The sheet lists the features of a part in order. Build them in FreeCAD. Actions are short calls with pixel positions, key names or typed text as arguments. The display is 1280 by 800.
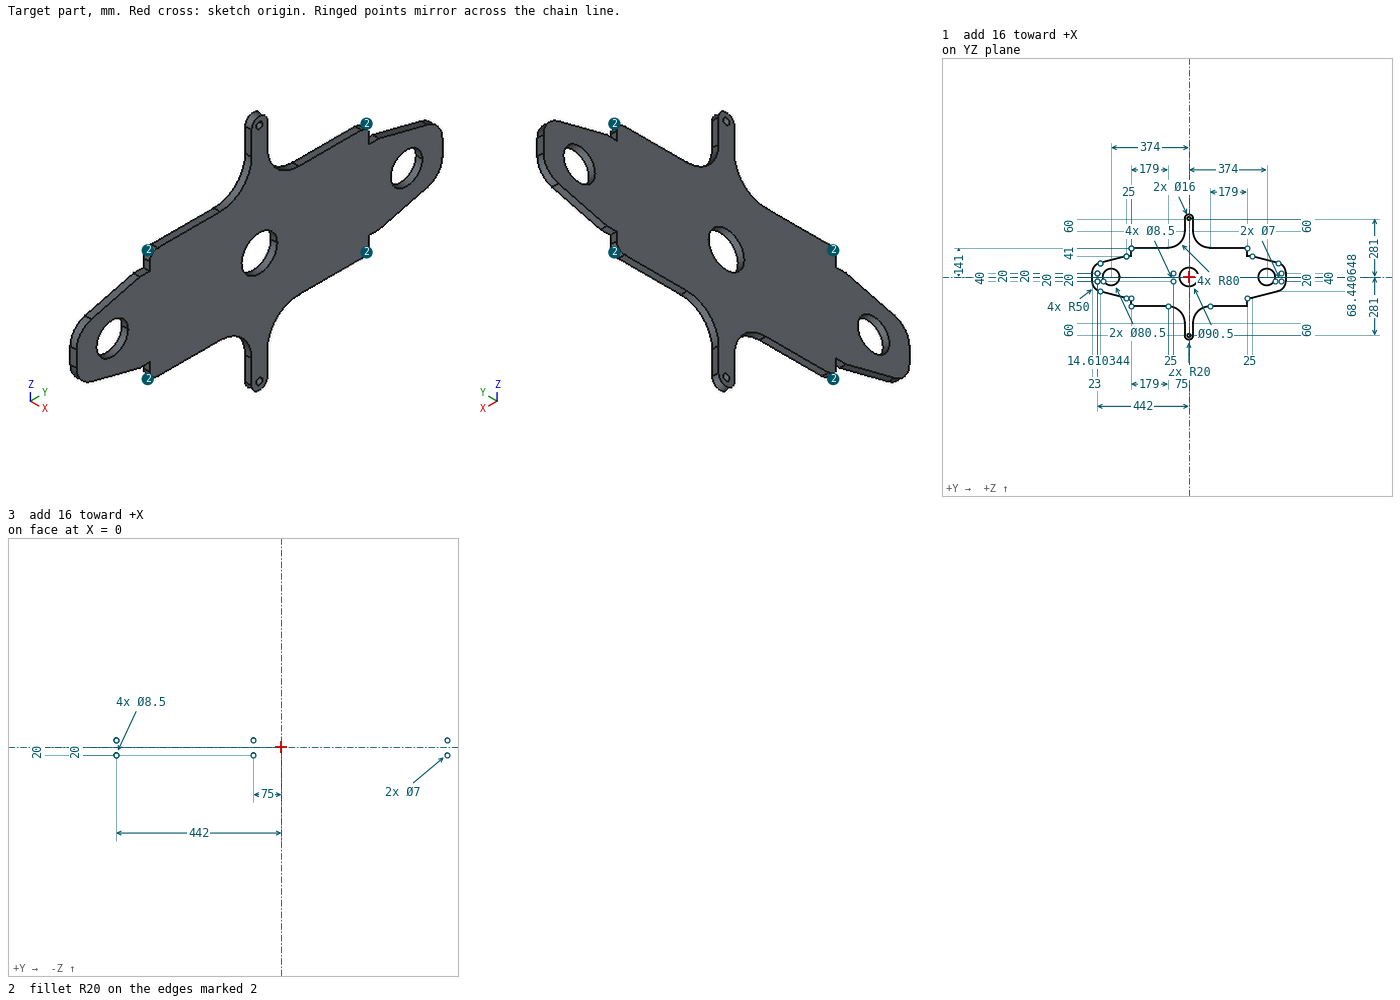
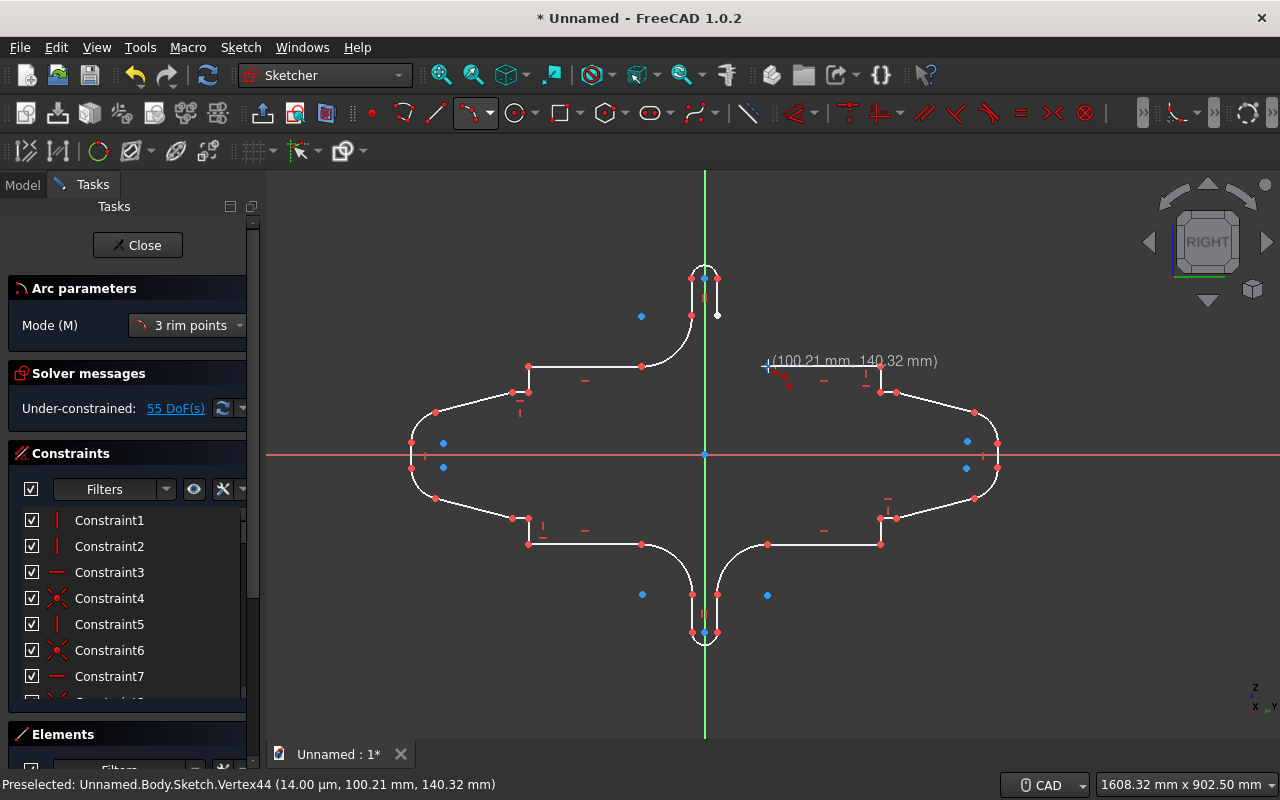
scroll(717, 315, up, 2)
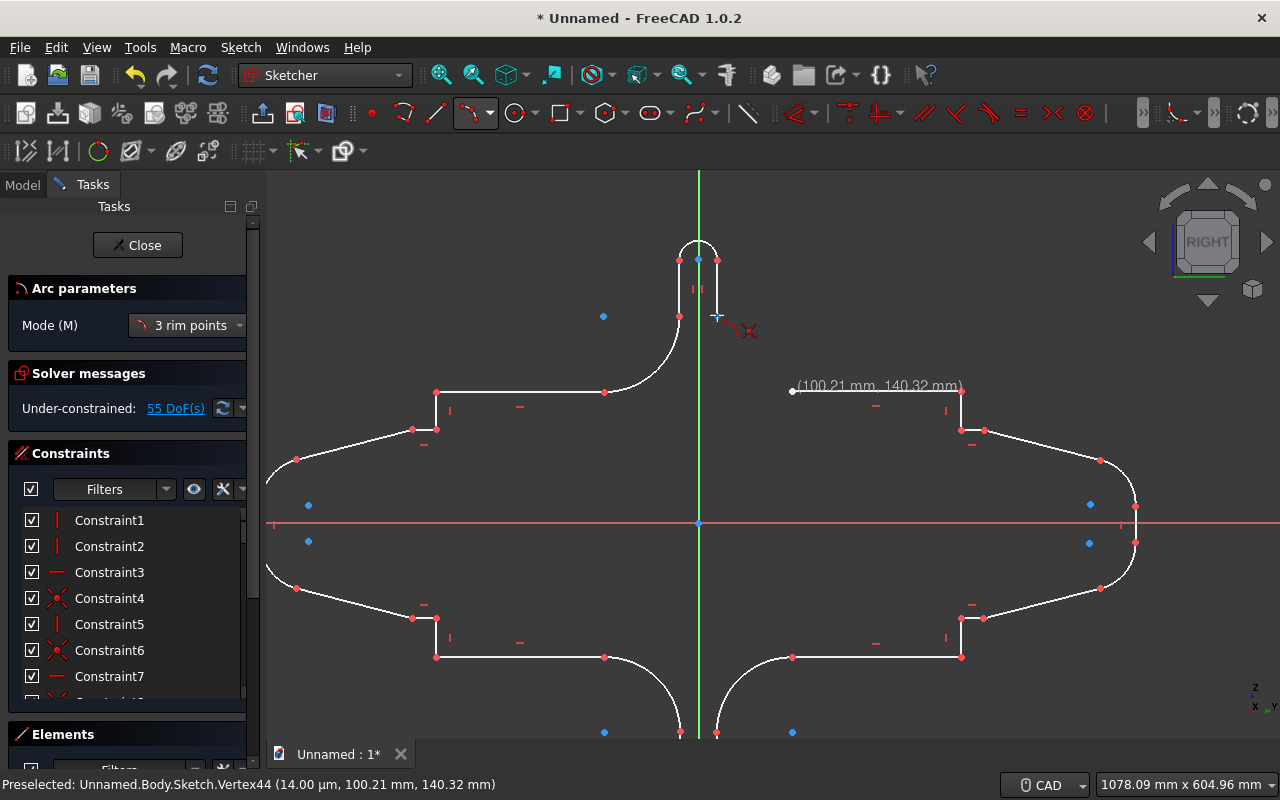
click(717, 316)
click(739, 369)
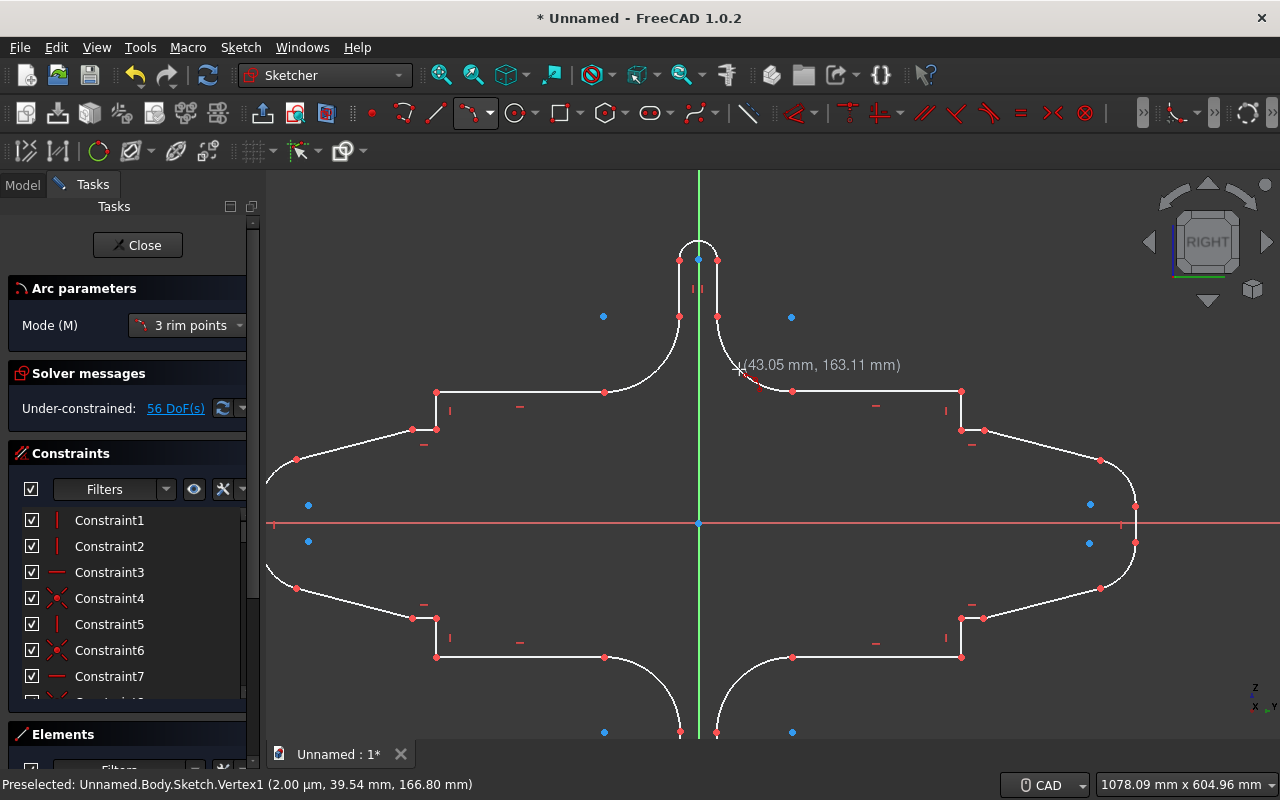
click(516, 114)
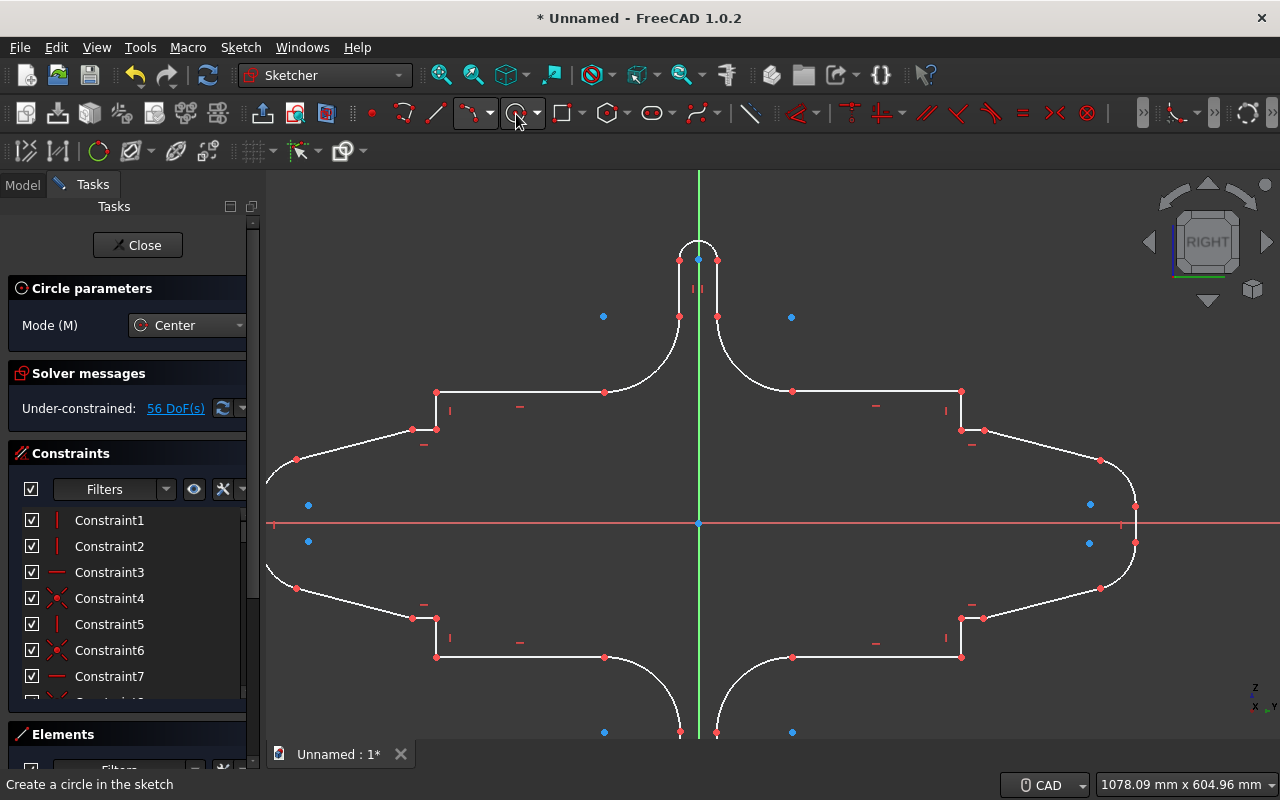
scroll(717, 314, down, 2)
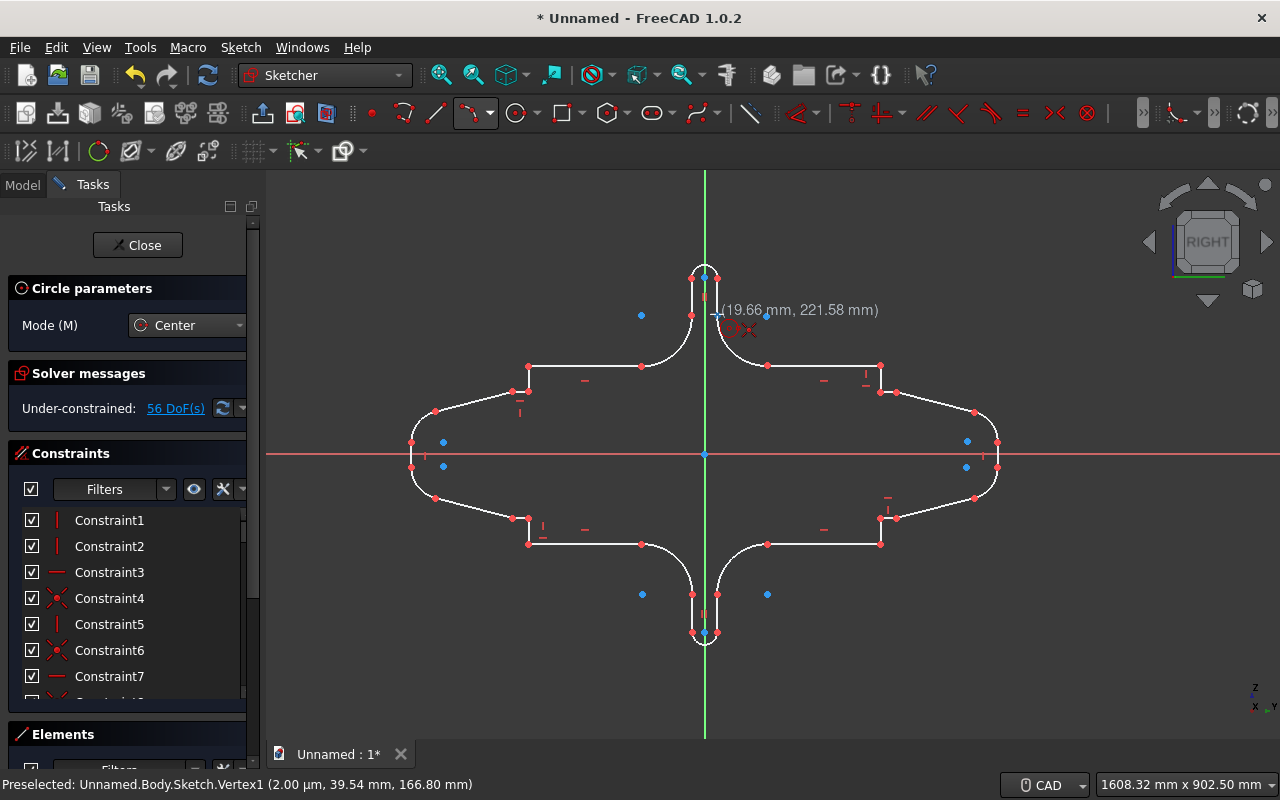
scroll(426, 467, up, 11)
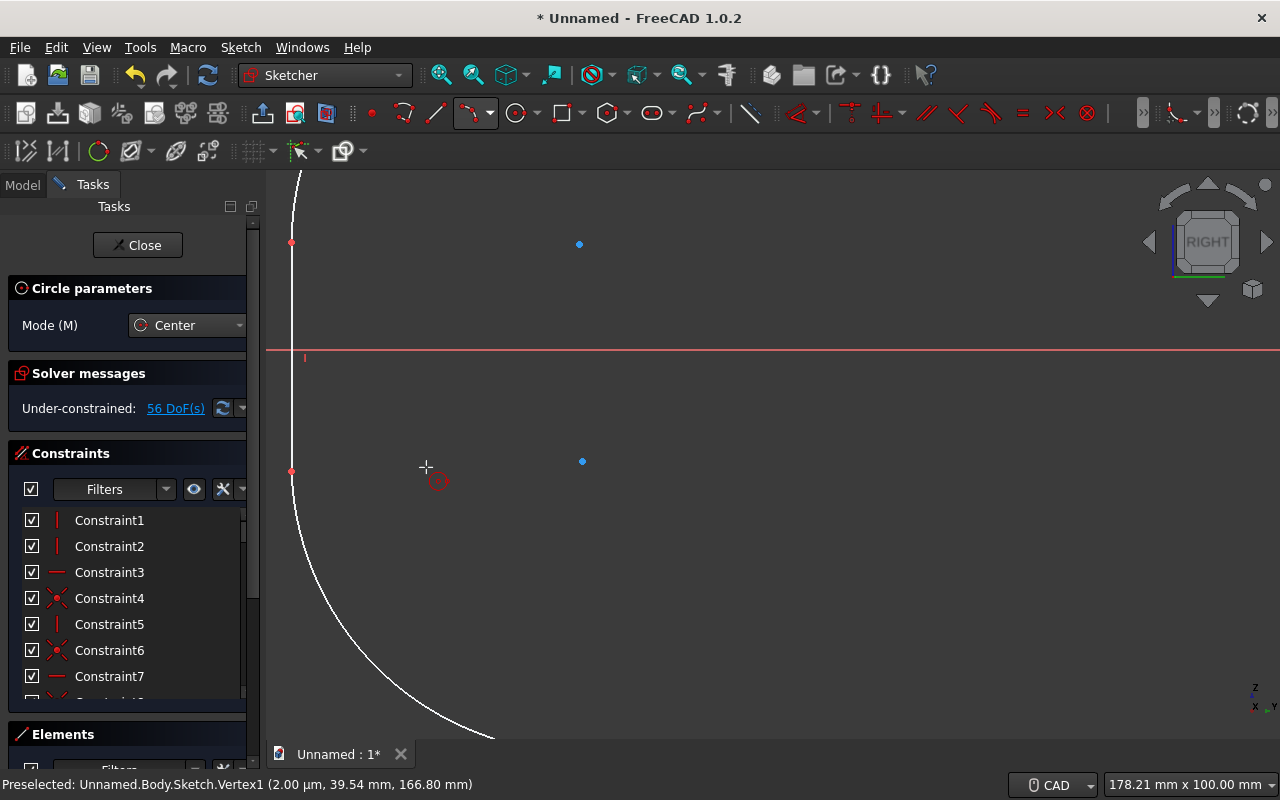
scroll(426, 468, down, 11)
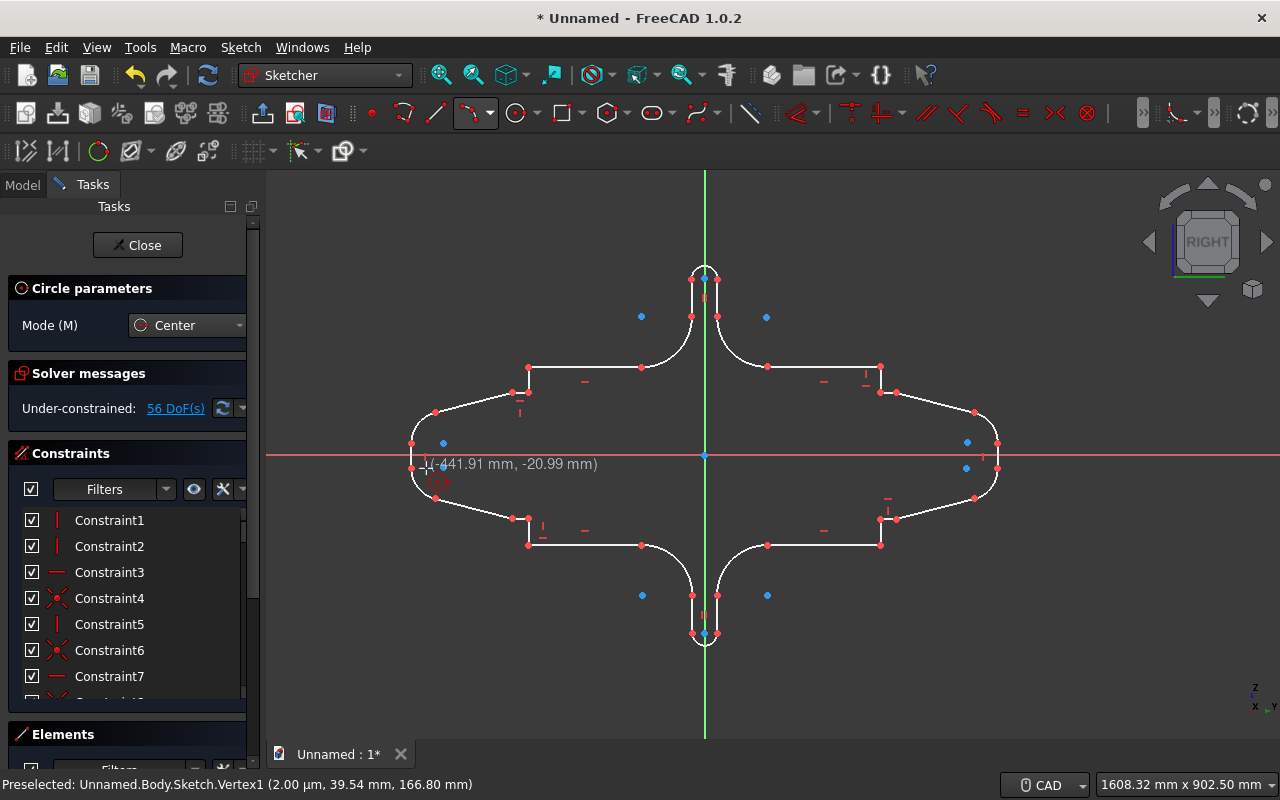
scroll(426, 468, up, 2)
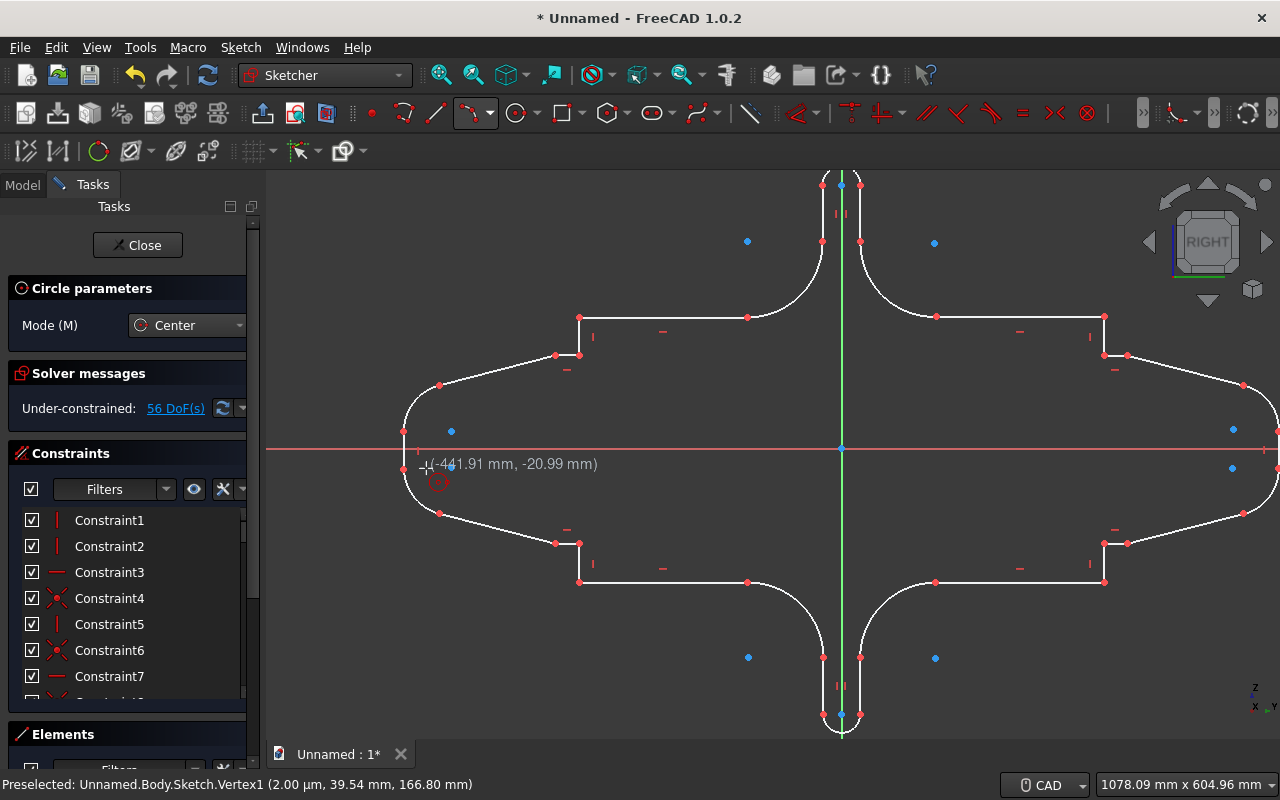
click(426, 468)
move(429, 465)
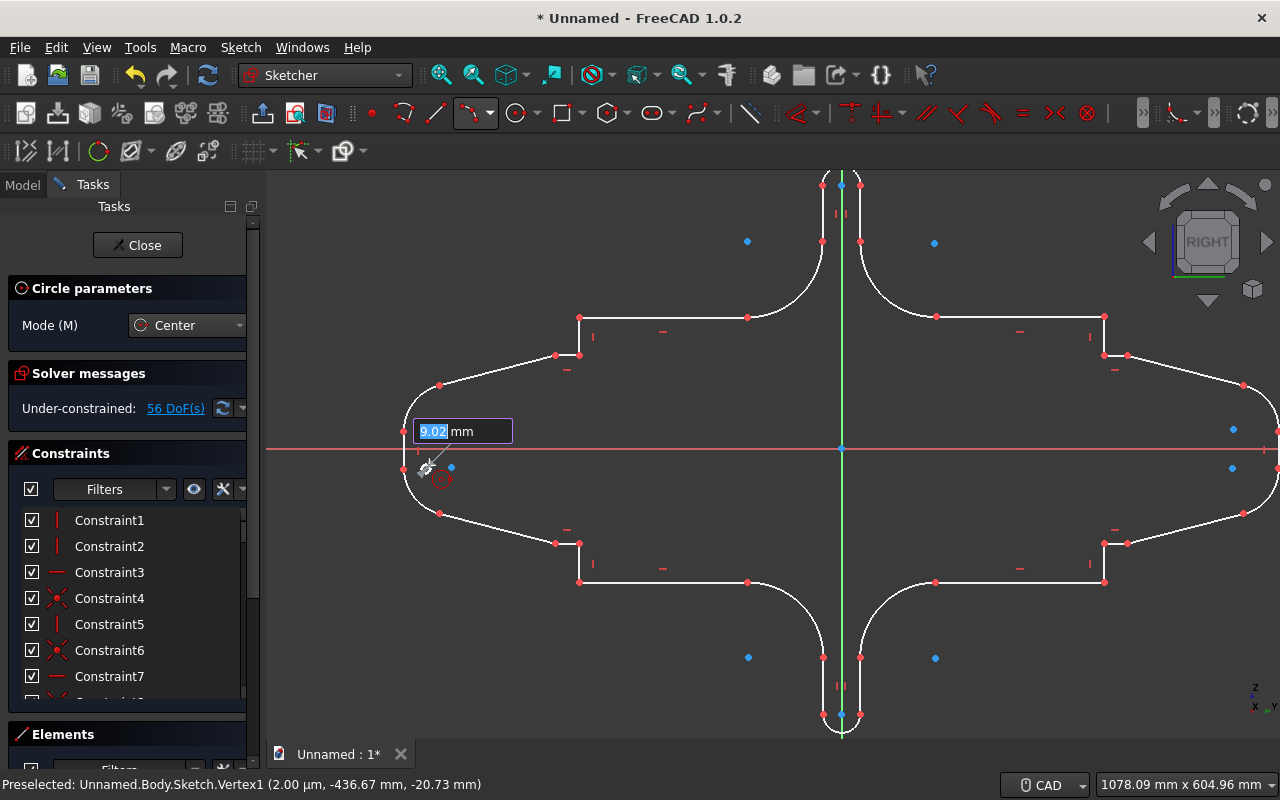
text(8.5)
key(Return)